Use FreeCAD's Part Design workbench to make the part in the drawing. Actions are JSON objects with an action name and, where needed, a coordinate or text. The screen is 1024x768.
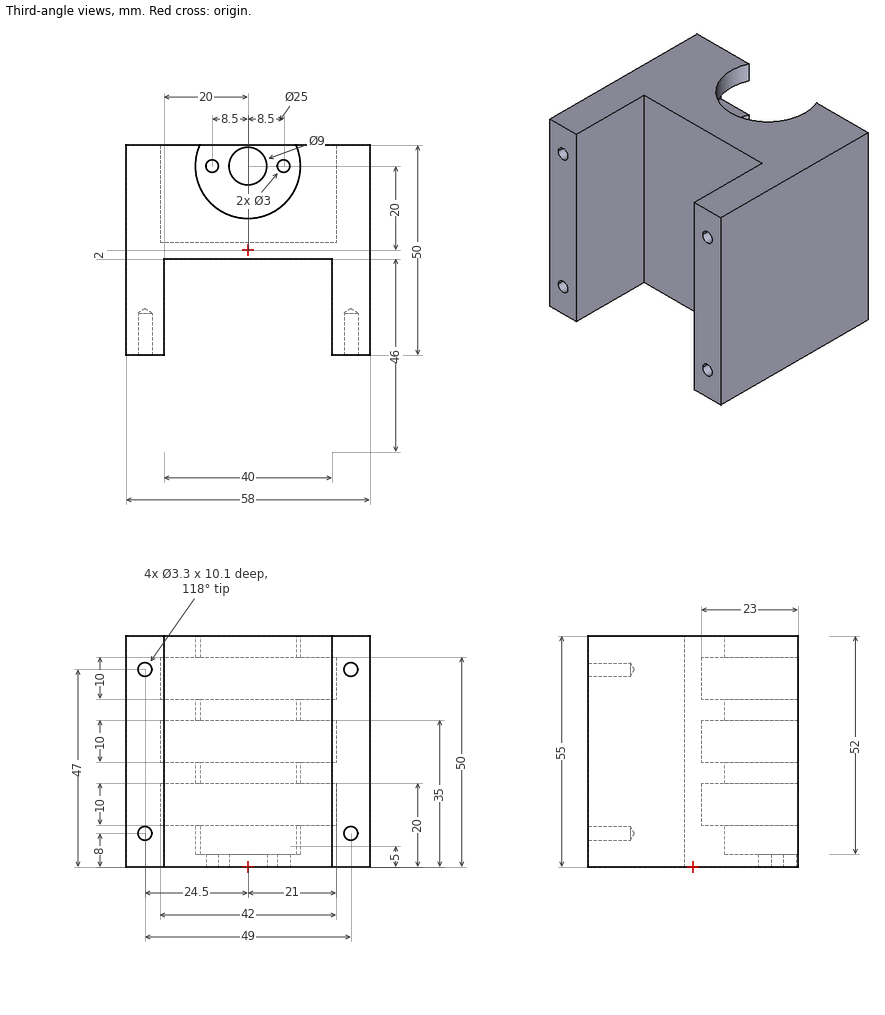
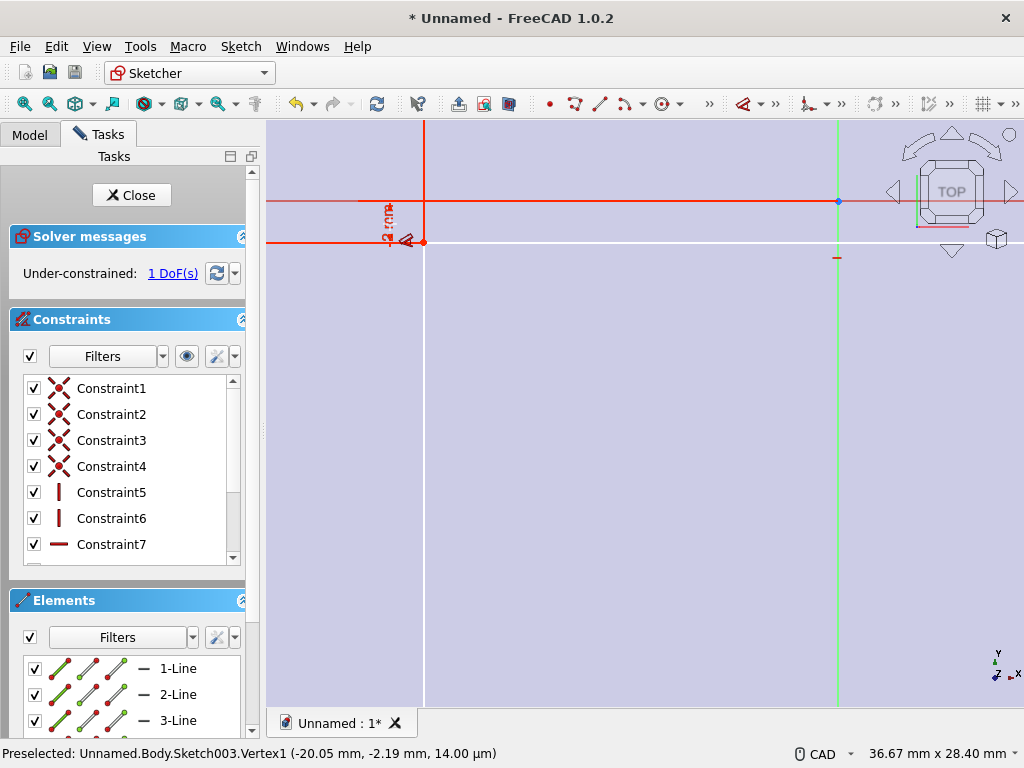
{"action": "left_click", "coordinate": [424, 243]}
{"action": "left_click", "coordinate": [631, 167]}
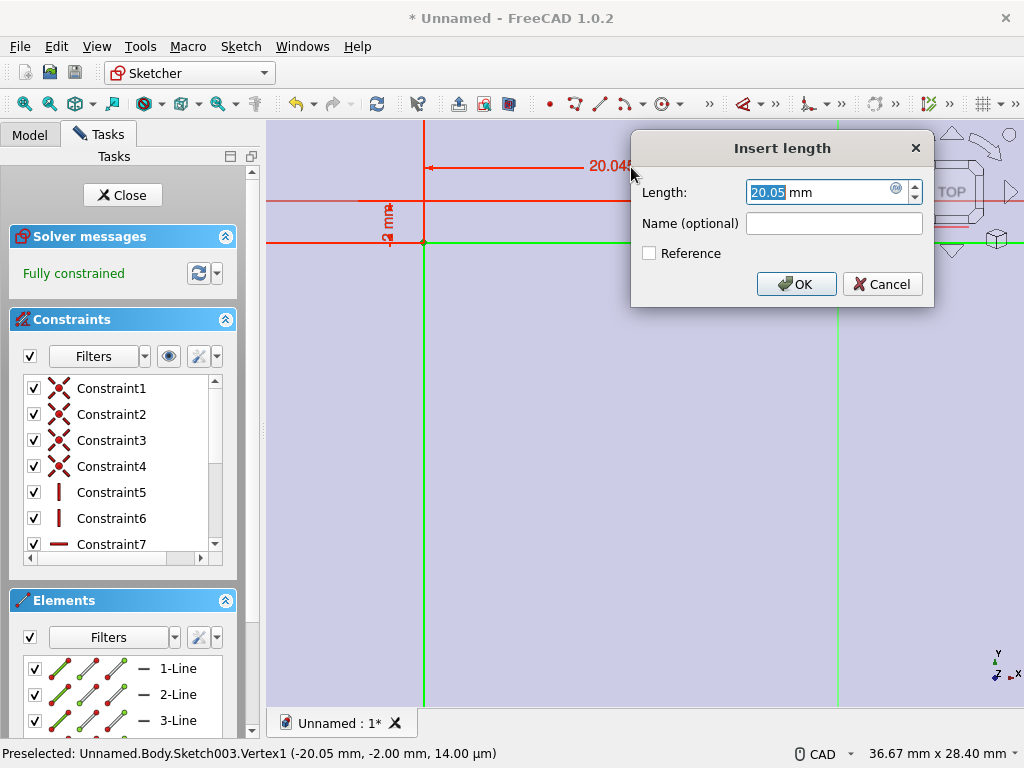
{"action": "type", "text": "20"}
{"action": "key", "text": "Return"}
{"action": "key", "text": "Escape"}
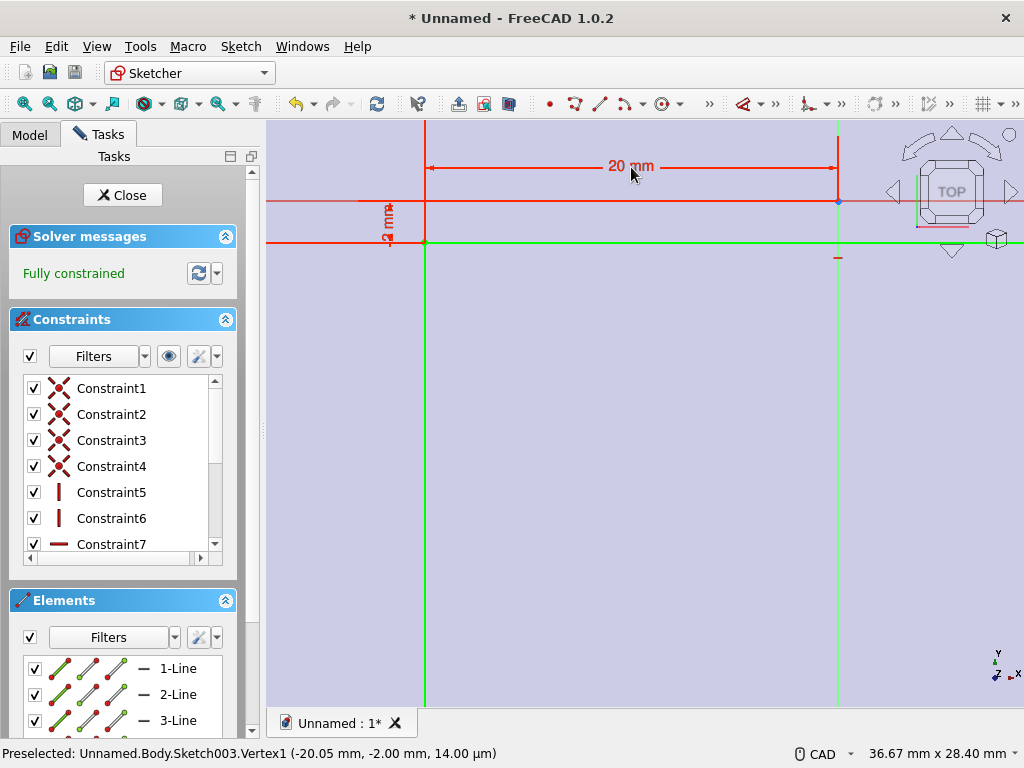
{"action": "left_click", "coordinate": [123, 195]}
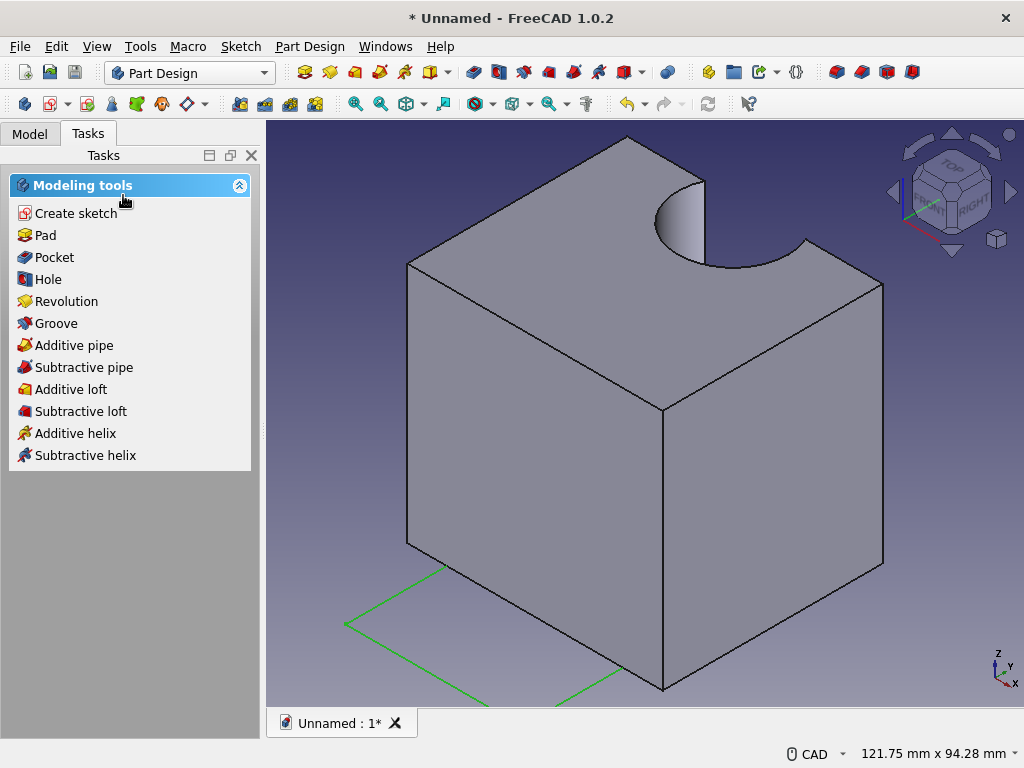
{"action": "left_click", "coordinate": [474, 72]}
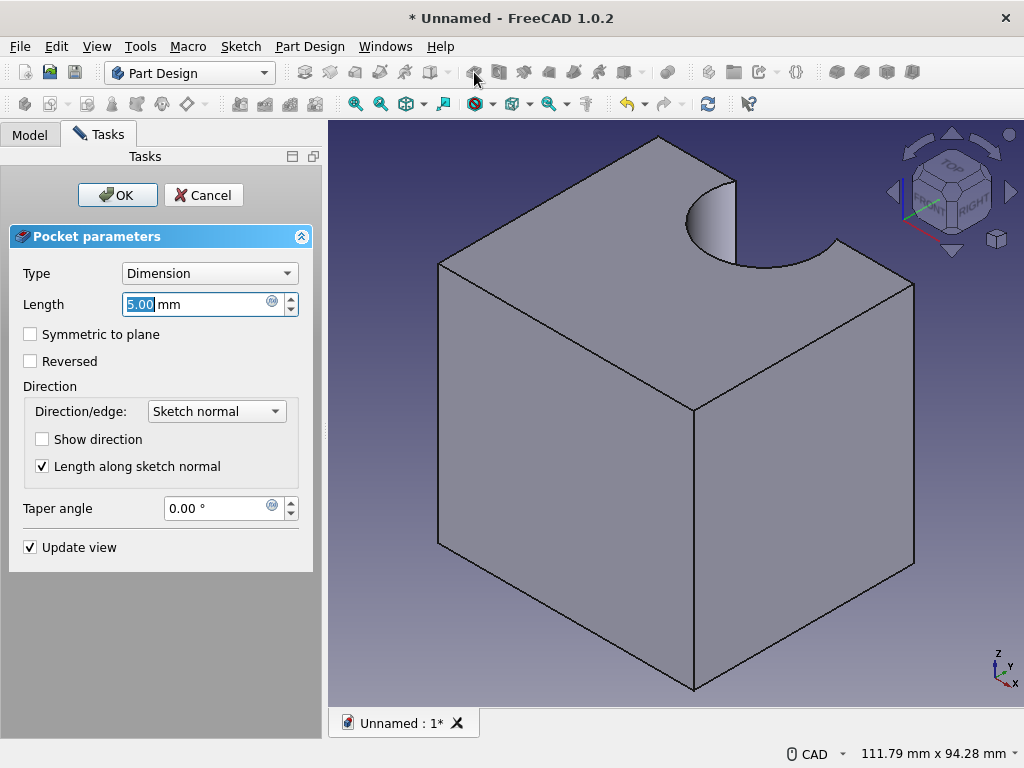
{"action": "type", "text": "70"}
{"action": "key", "text": "Tab"}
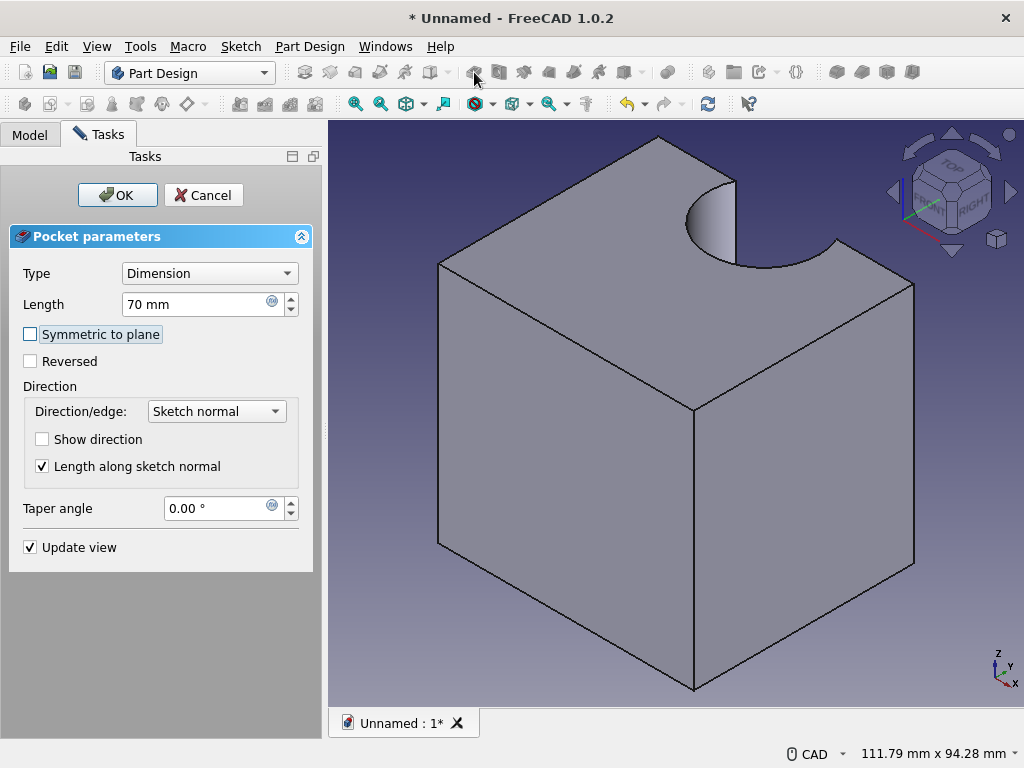
{"action": "left_click", "coordinate": [31, 361]}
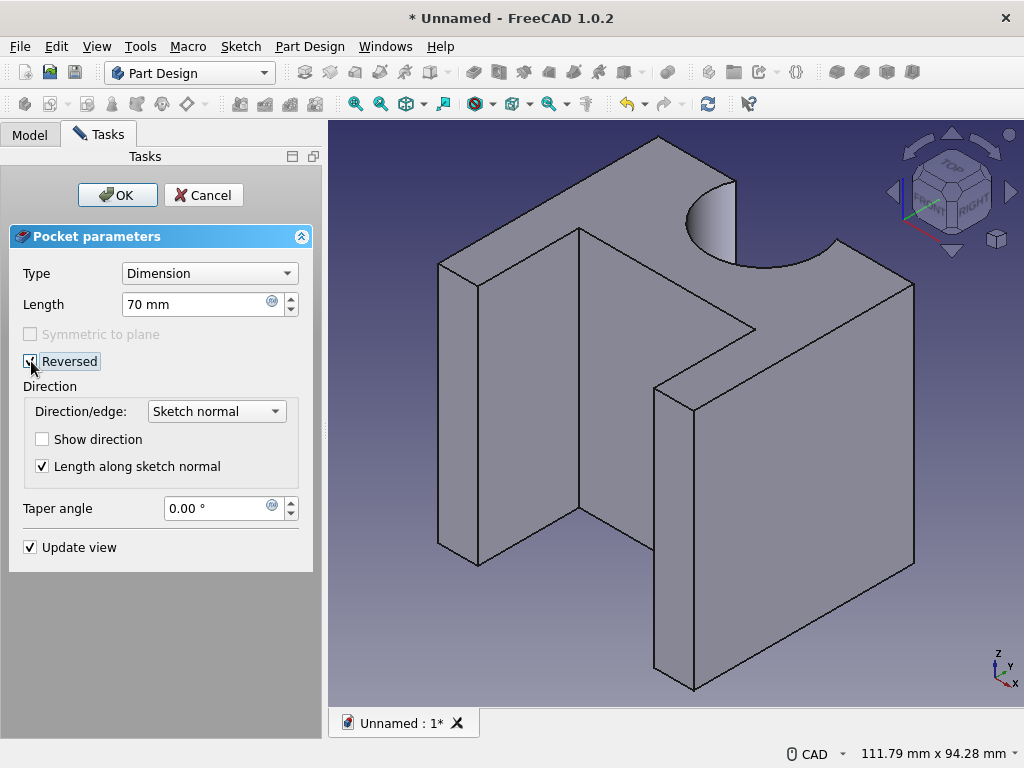
{"action": "left_click", "coordinate": [118, 195]}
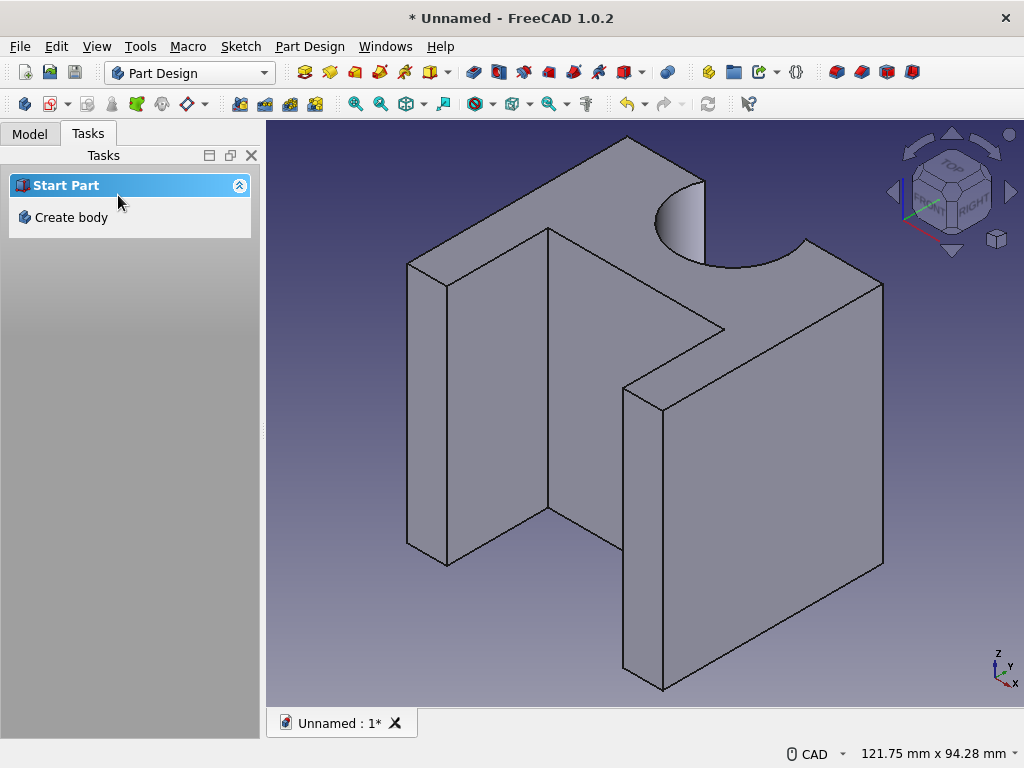
{"action": "left_click", "coordinate": [643, 458]}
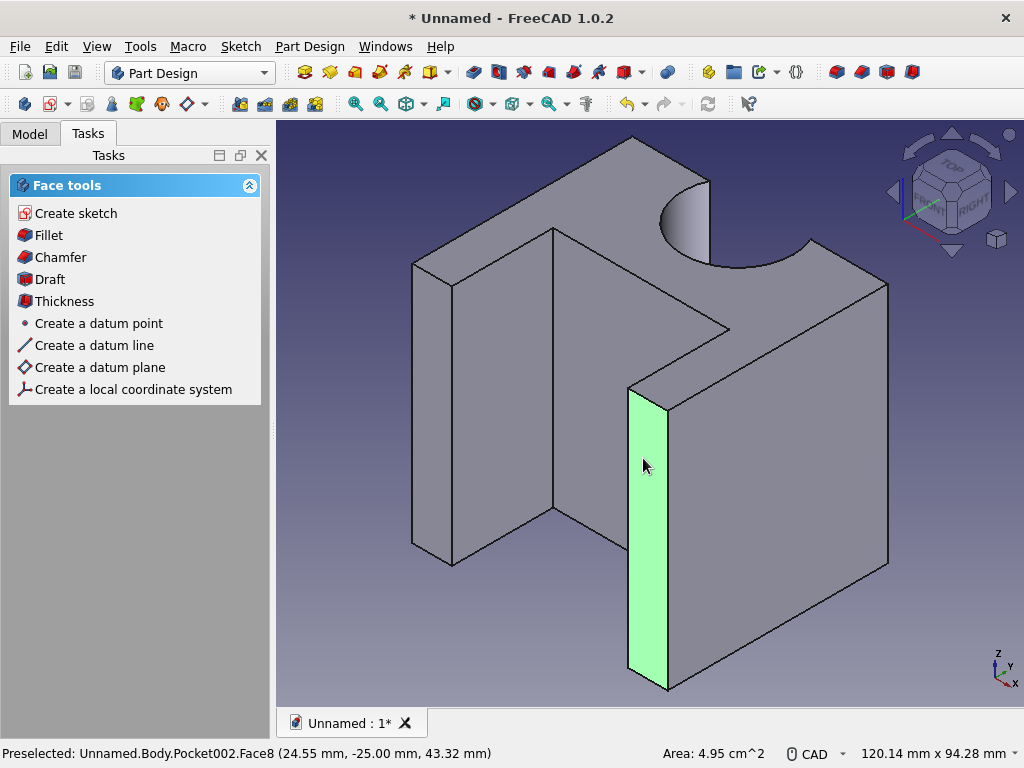
{"action": "left_click", "coordinate": [50, 104]}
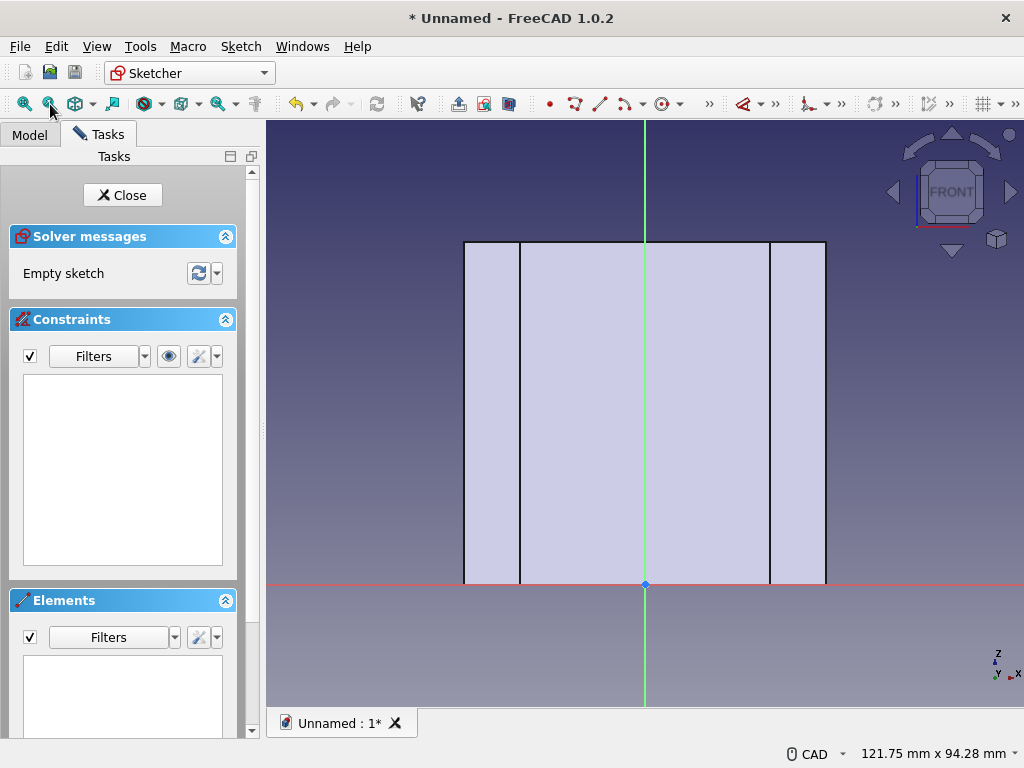
{"action": "left_click", "coordinate": [662, 104]}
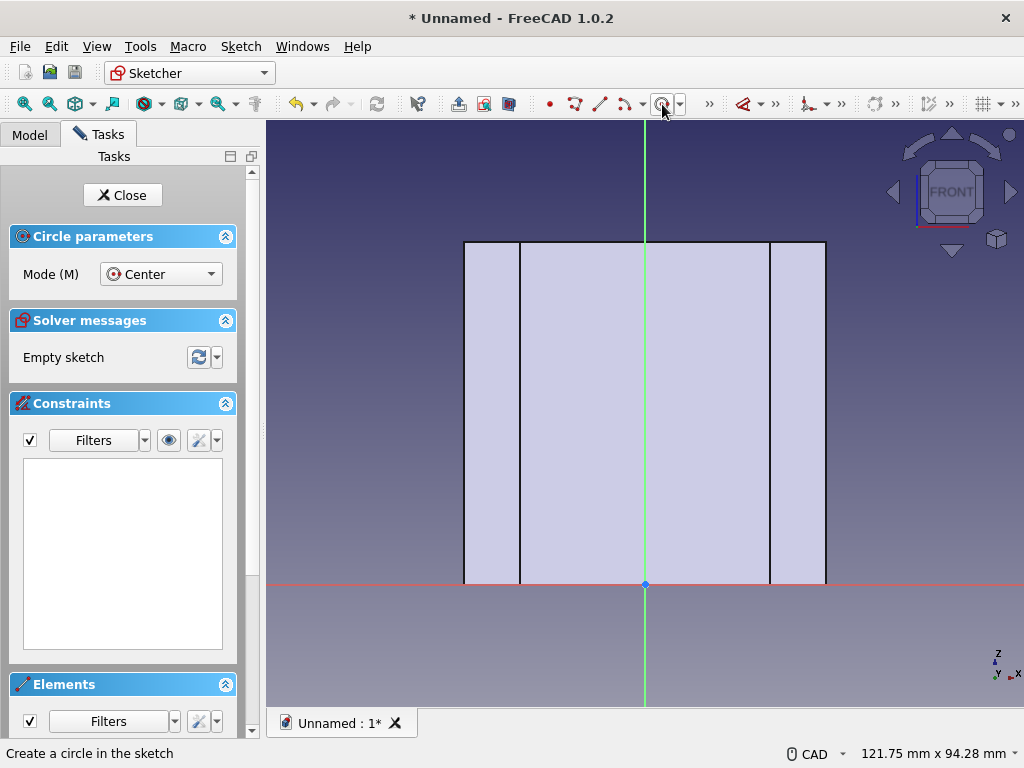
{"action": "scroll", "coordinate": [492, 292], "scroll_direction": "up", "scroll_amount": 4}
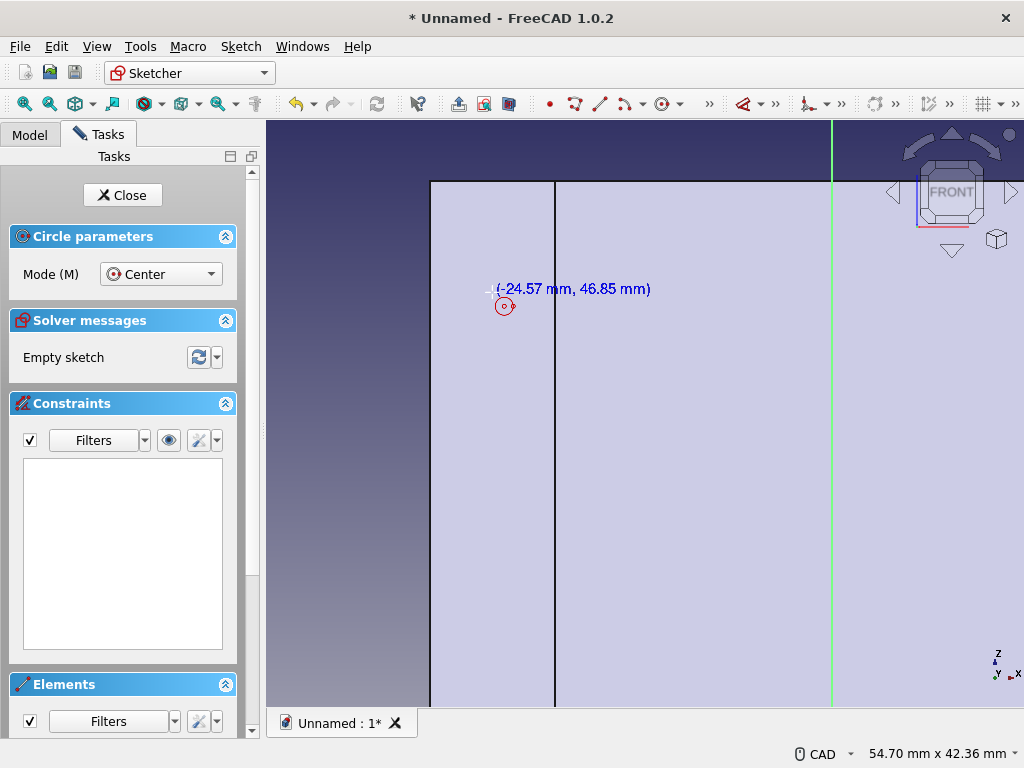
{"action": "left_click", "coordinate": [493, 292]}
{"action": "mouse_move", "coordinate": [509, 276]}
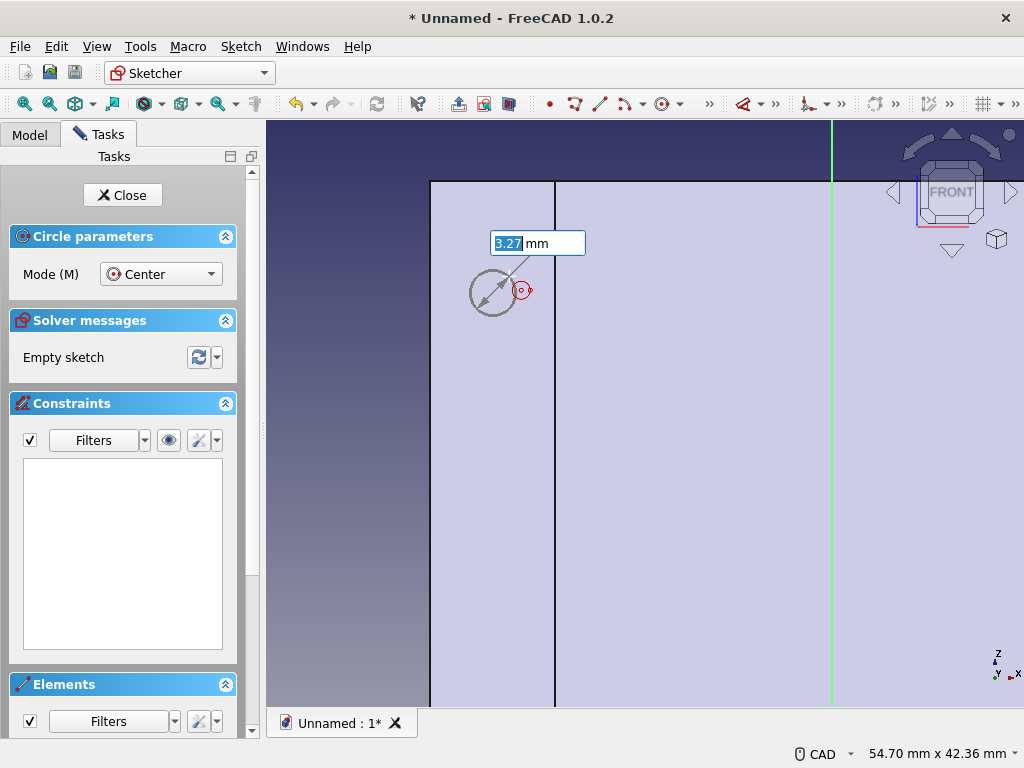
{"action": "type", "text": "3.3"}
{"action": "key", "text": "Return"}